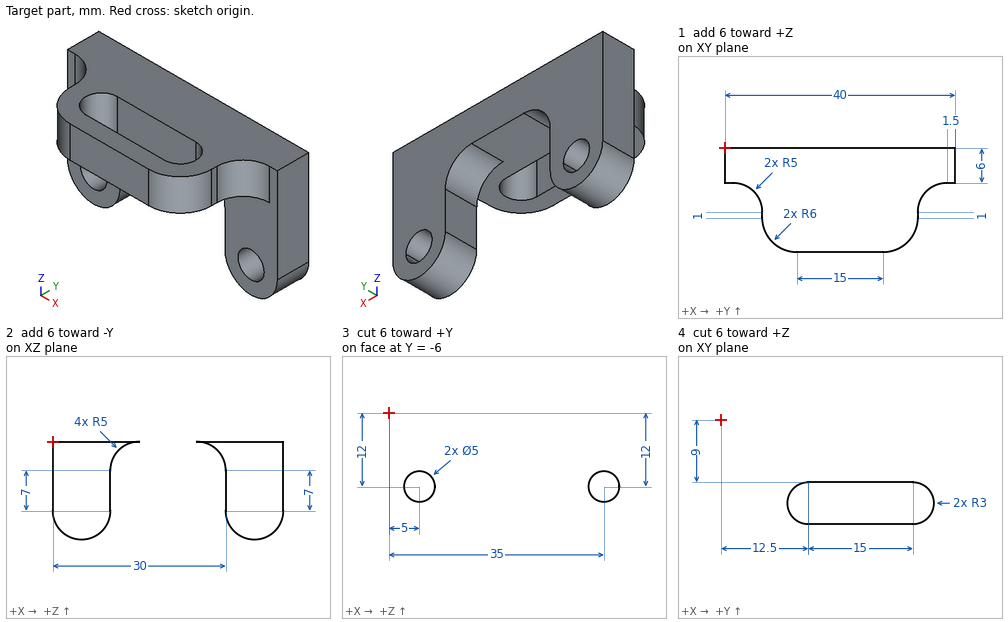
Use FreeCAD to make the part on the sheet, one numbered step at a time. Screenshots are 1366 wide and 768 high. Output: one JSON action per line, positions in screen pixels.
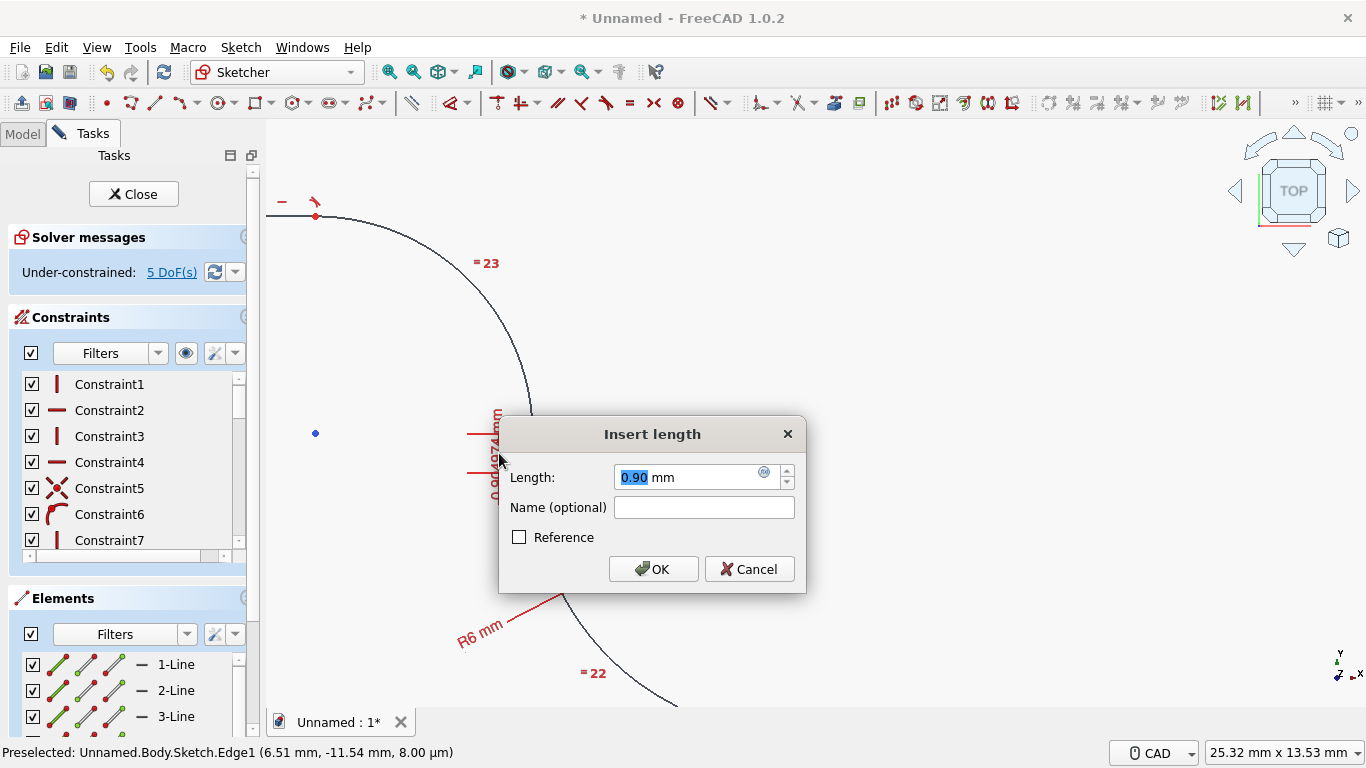
{"action": "type", "text": "1"}
{"action": "key", "text": "Return"}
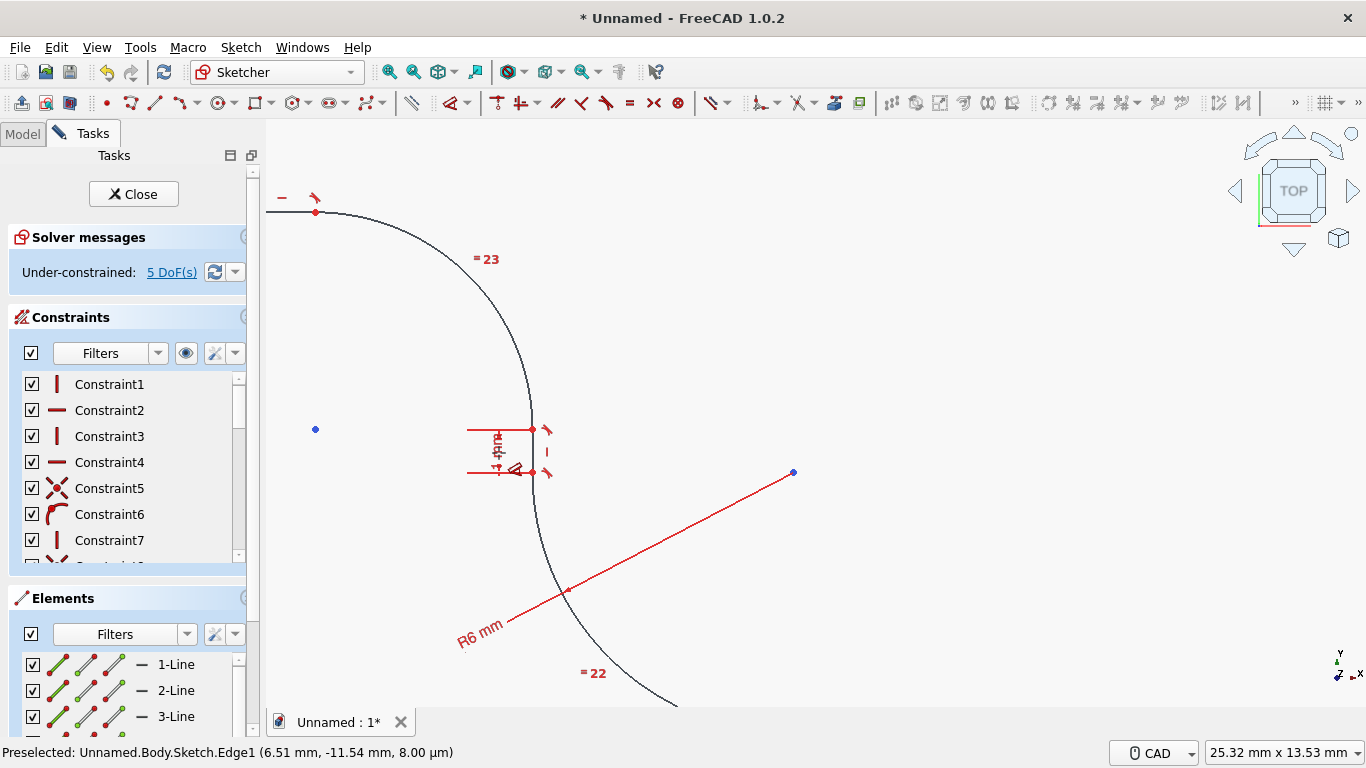
{"action": "scroll", "coordinate": [532, 453], "scroll_direction": "down", "scroll_amount": 5}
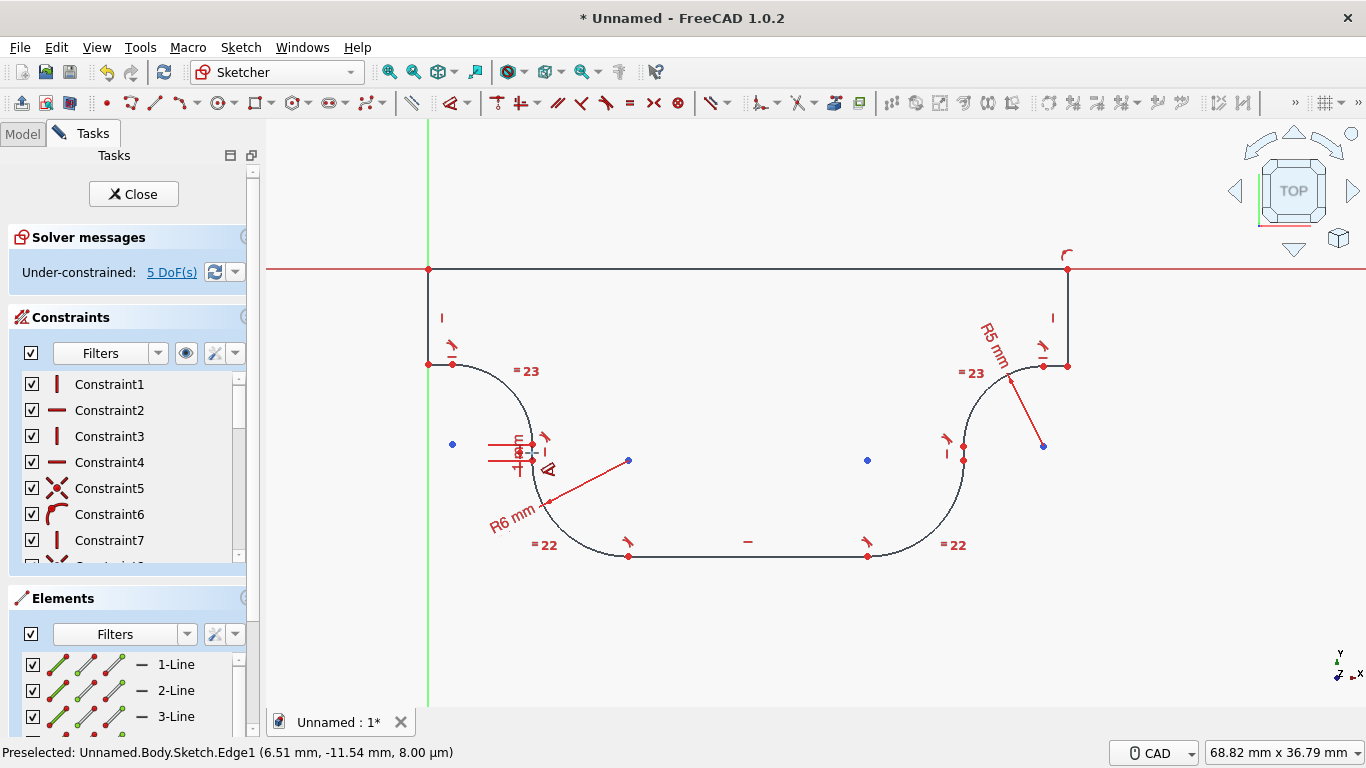
{"action": "scroll", "coordinate": [964, 456], "scroll_direction": "up", "scroll_amount": 6}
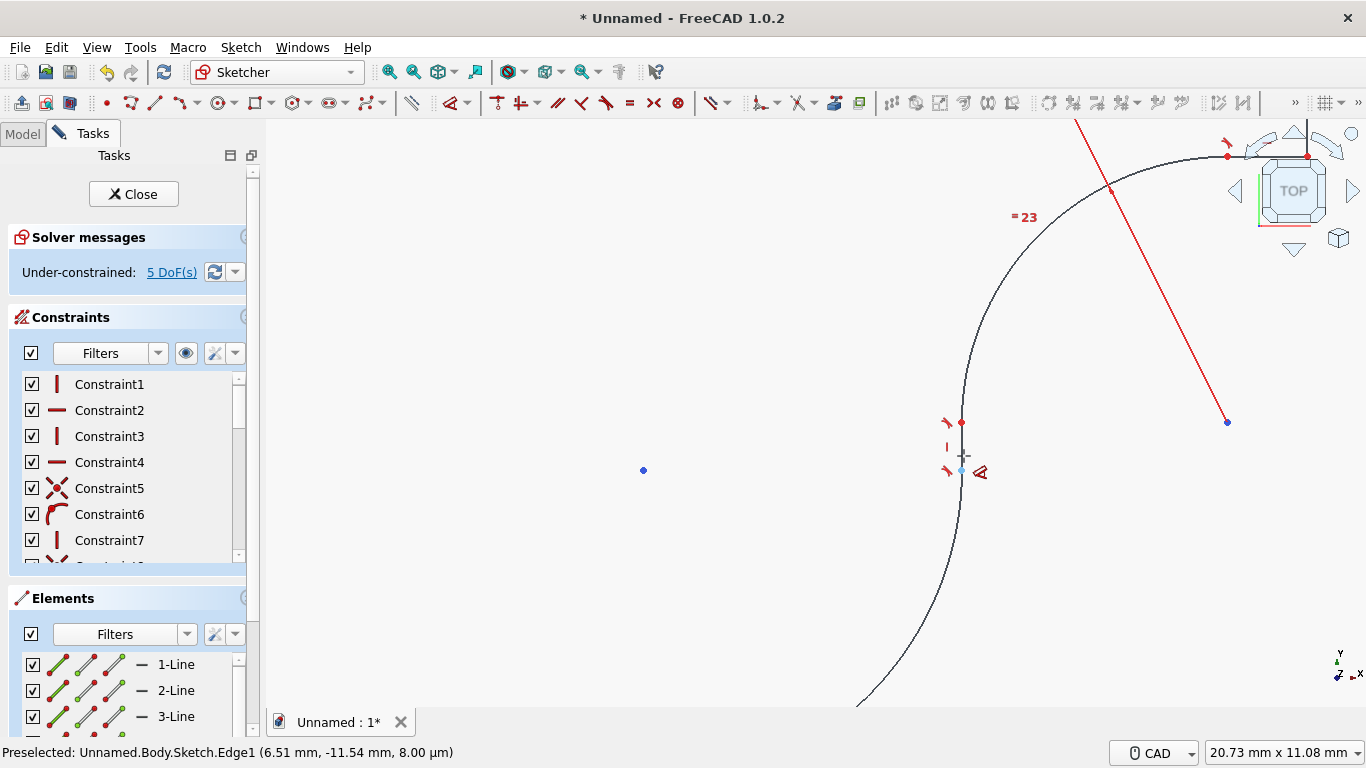
{"action": "left_click", "coordinate": [962, 456]}
{"action": "left_click", "coordinate": [996, 446]}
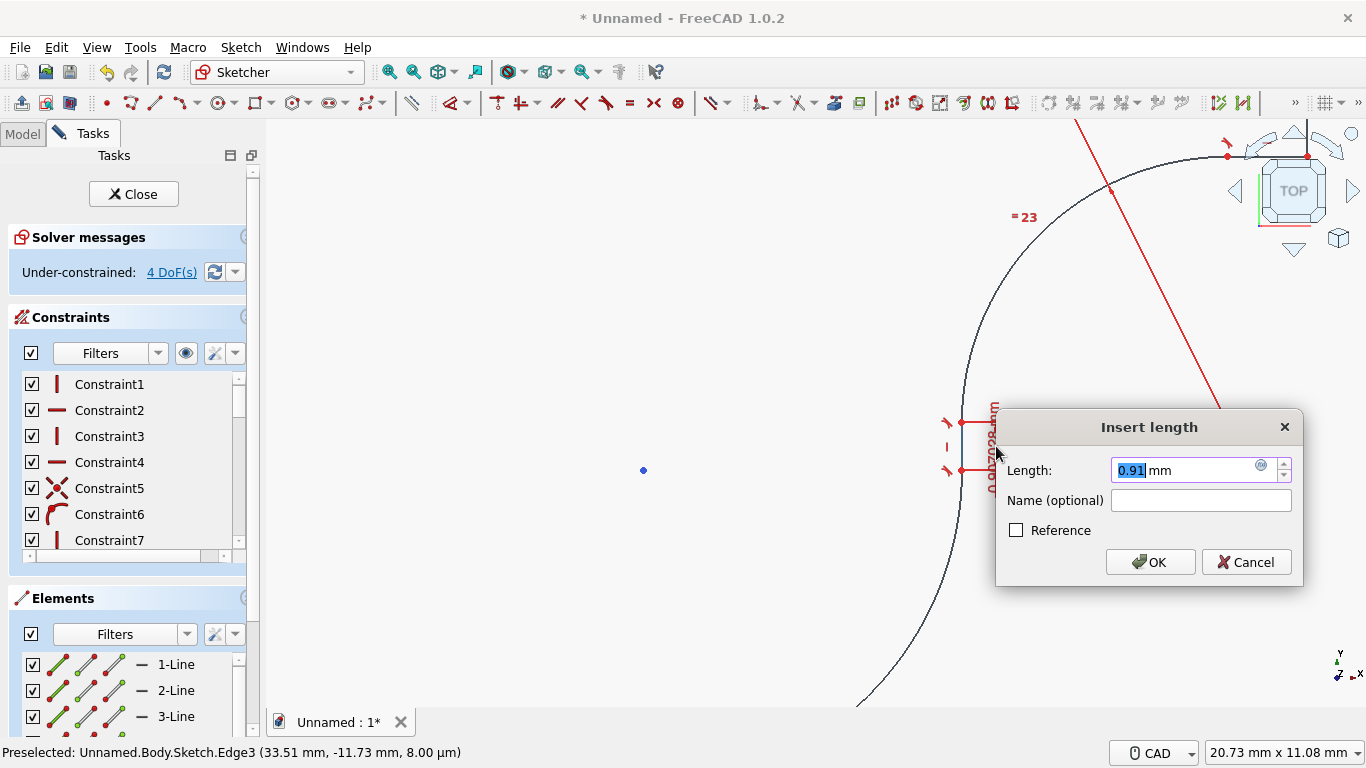
{"action": "type", "text": "1"}
{"action": "key", "text": "Return"}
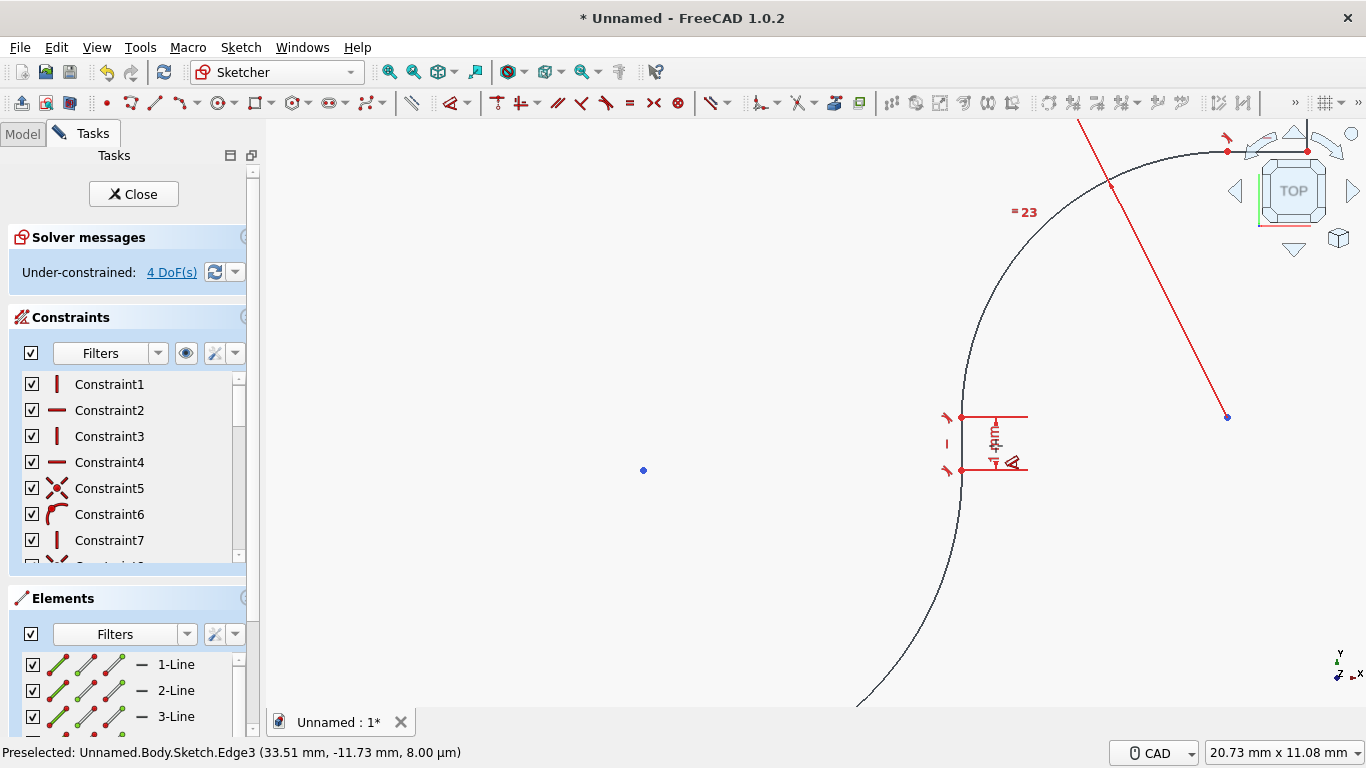
{"action": "scroll", "coordinate": [964, 456], "scroll_direction": "down", "scroll_amount": 6}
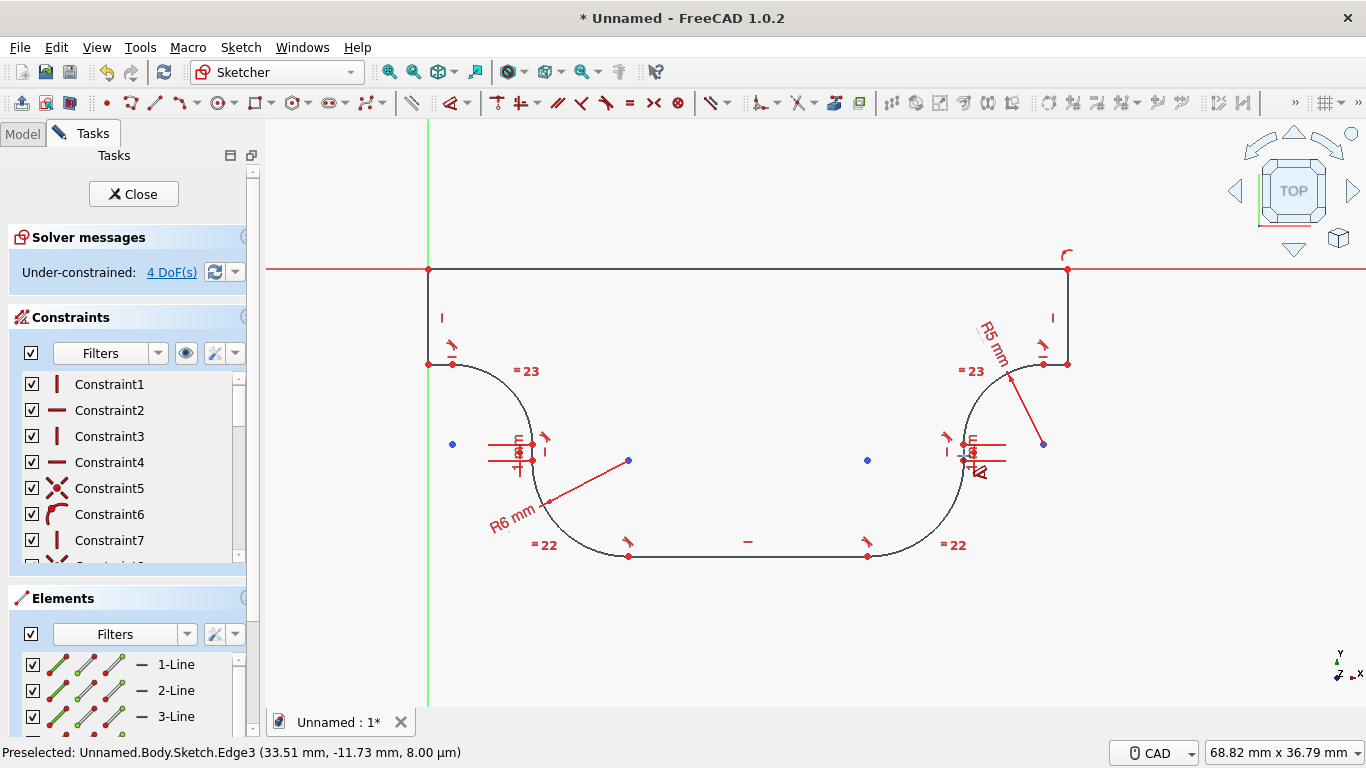
{"action": "left_click", "coordinate": [1068, 336]}
{"action": "left_click", "coordinate": [1102, 317]}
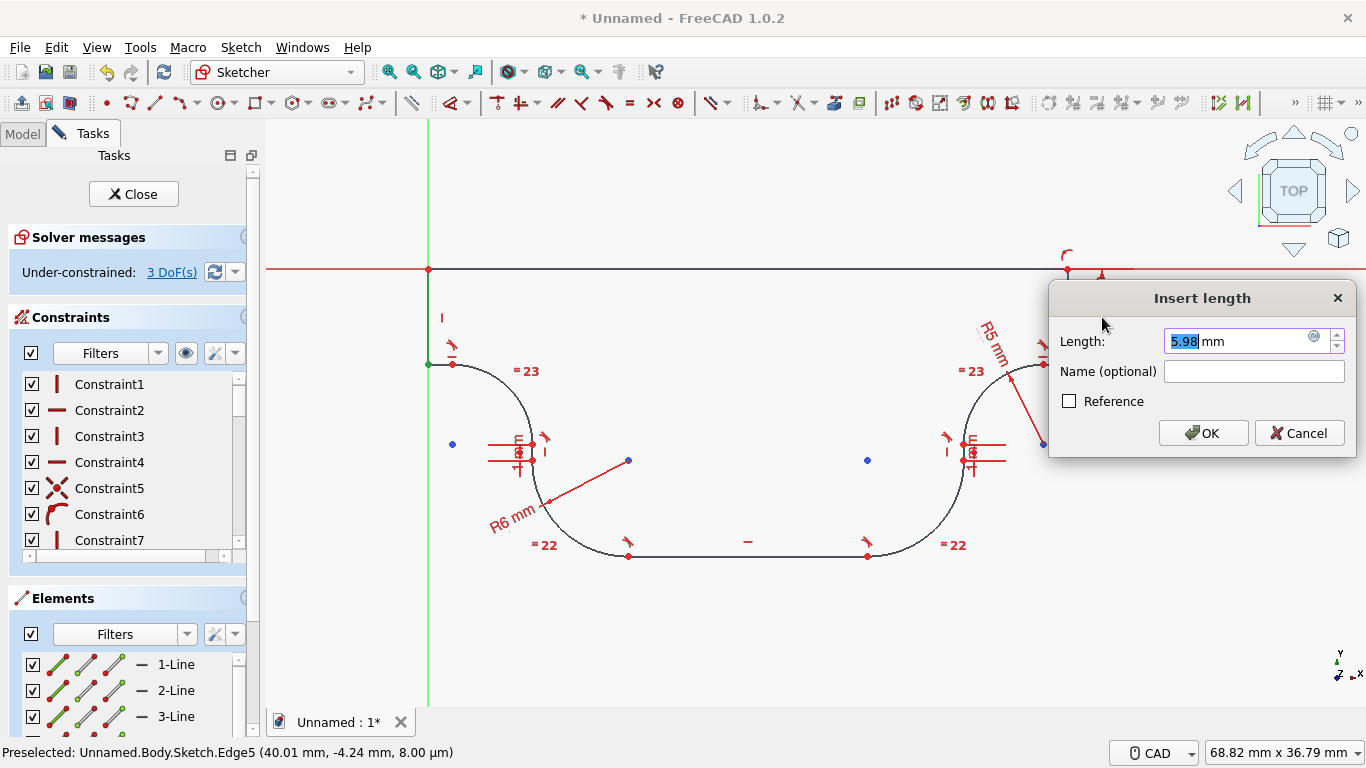
{"action": "type", "text": "6"}
{"action": "key", "text": "Return"}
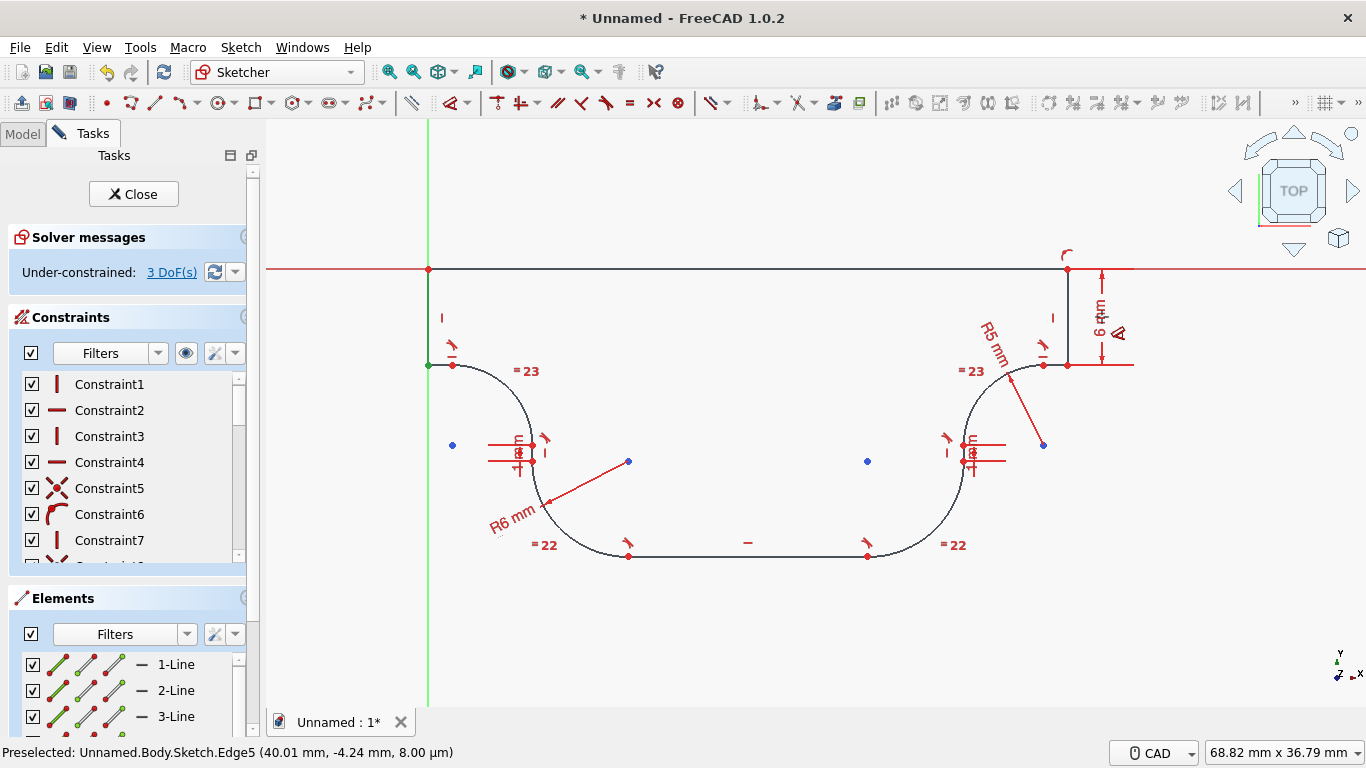
{"action": "left_click", "coordinate": [700, 557]}
{"action": "left_click", "coordinate": [748, 591]}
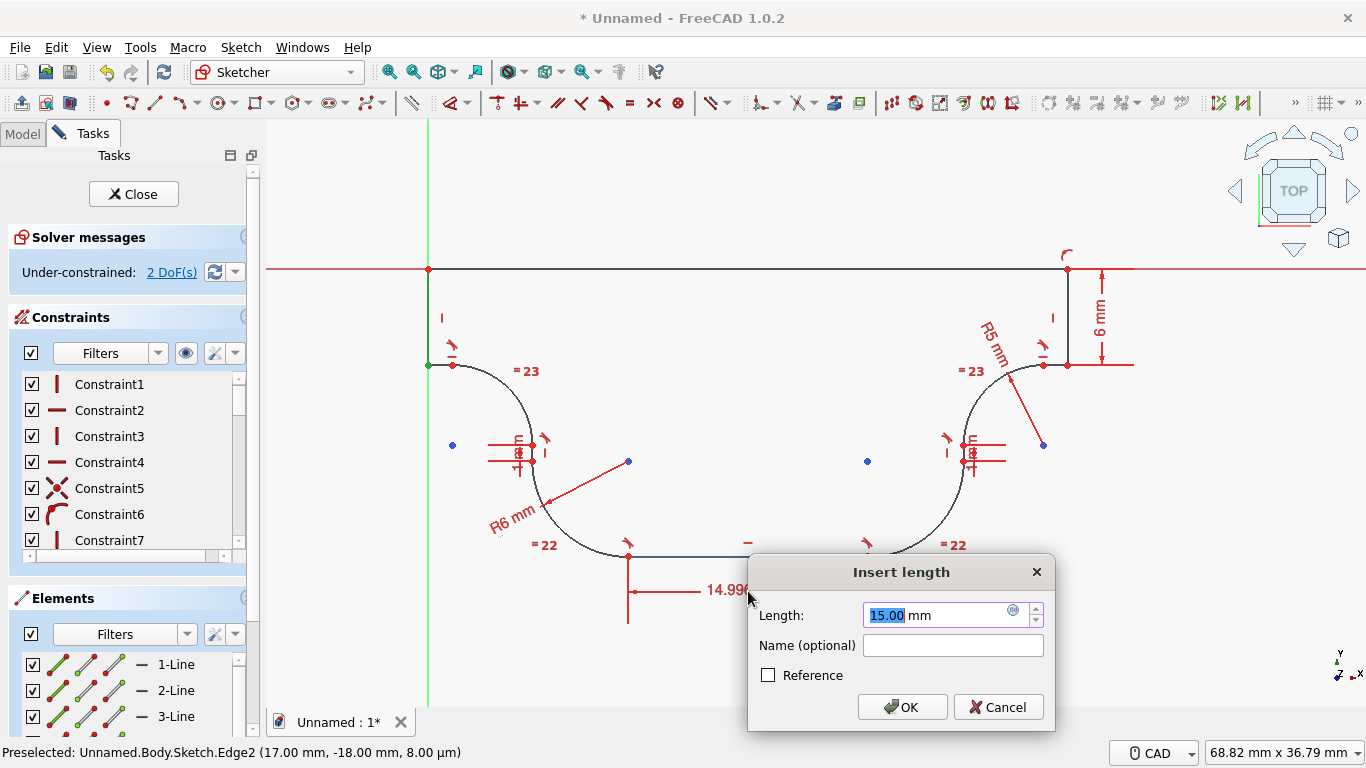
{"action": "type", "text": "15"}
{"action": "key", "text": "Return"}